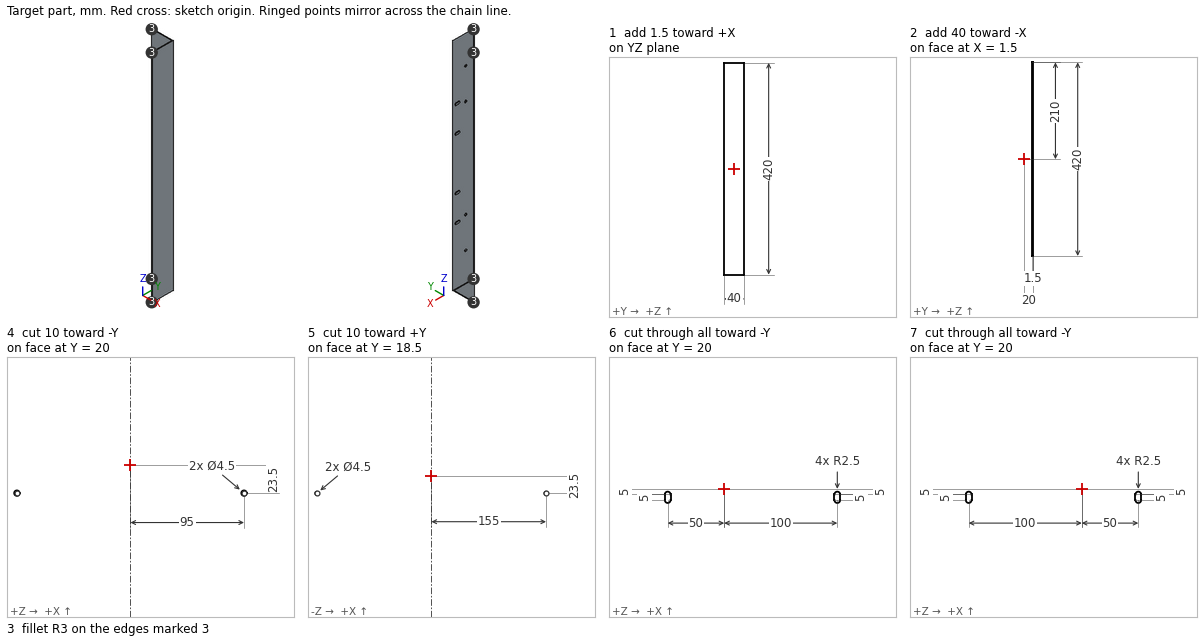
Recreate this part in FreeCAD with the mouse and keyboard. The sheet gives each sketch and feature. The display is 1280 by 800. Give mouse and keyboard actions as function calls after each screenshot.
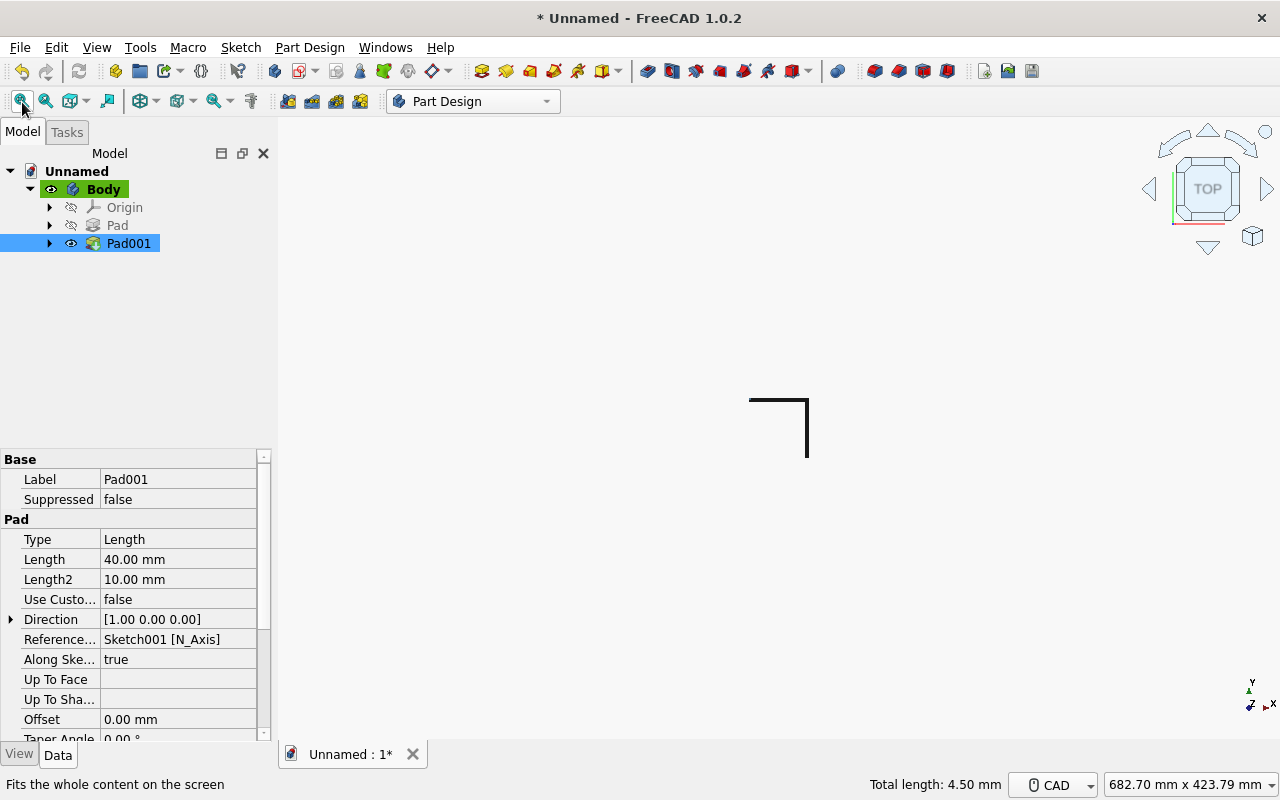
click(22, 102)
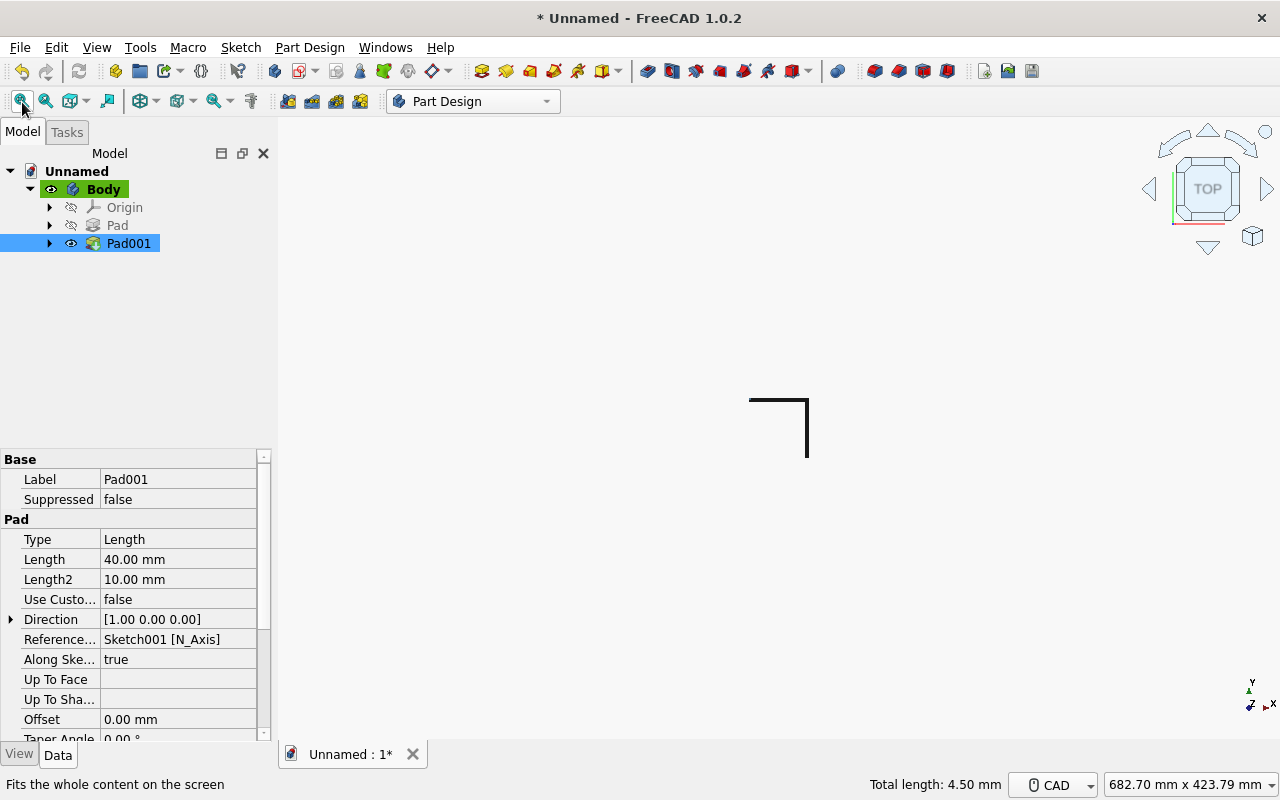
scroll(807, 456, up, 15)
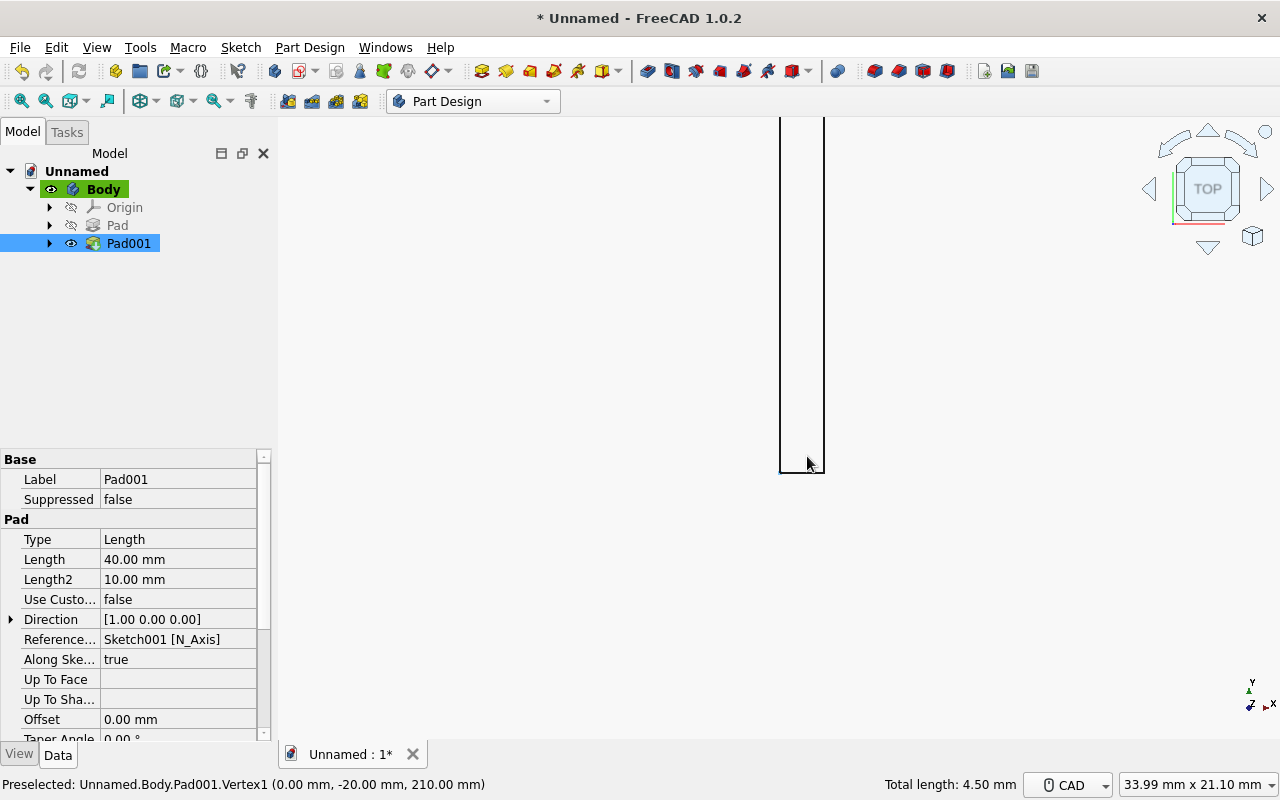
click(802, 472, ctrl)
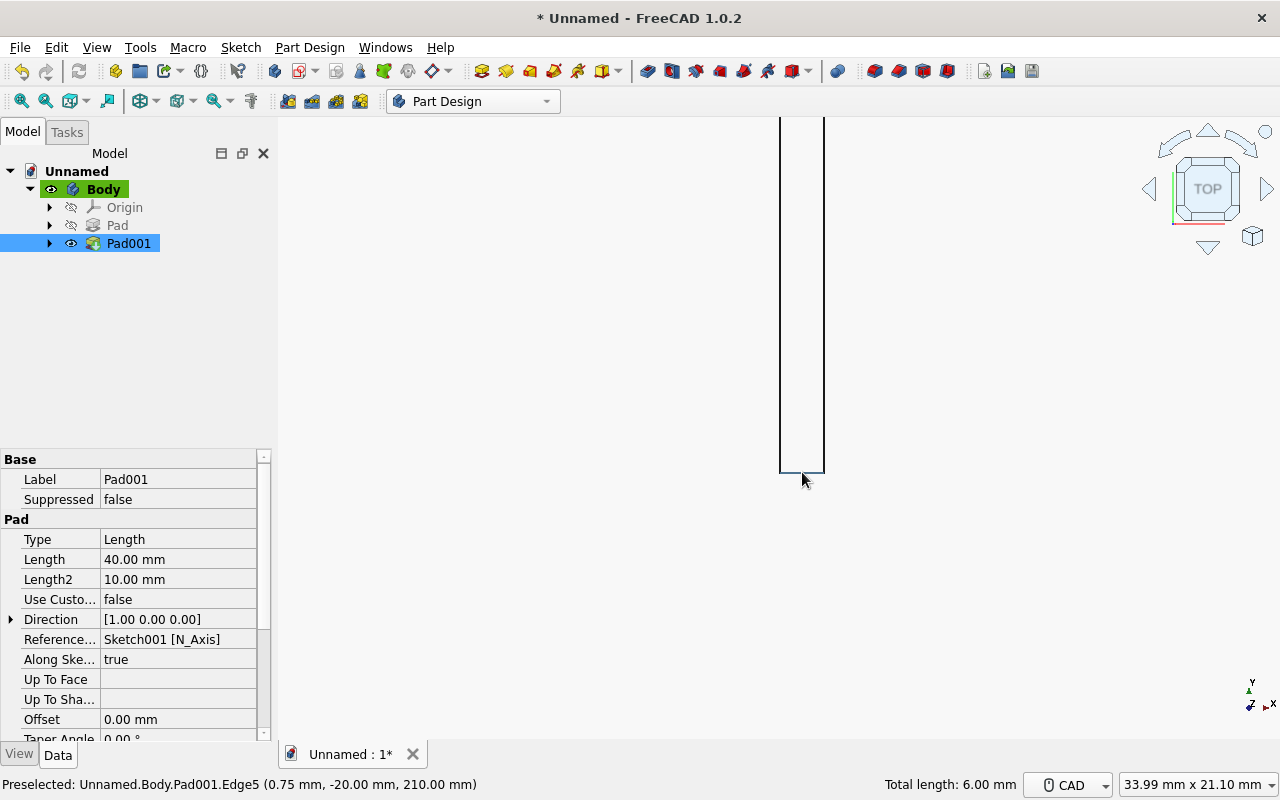
key(v)
key(1)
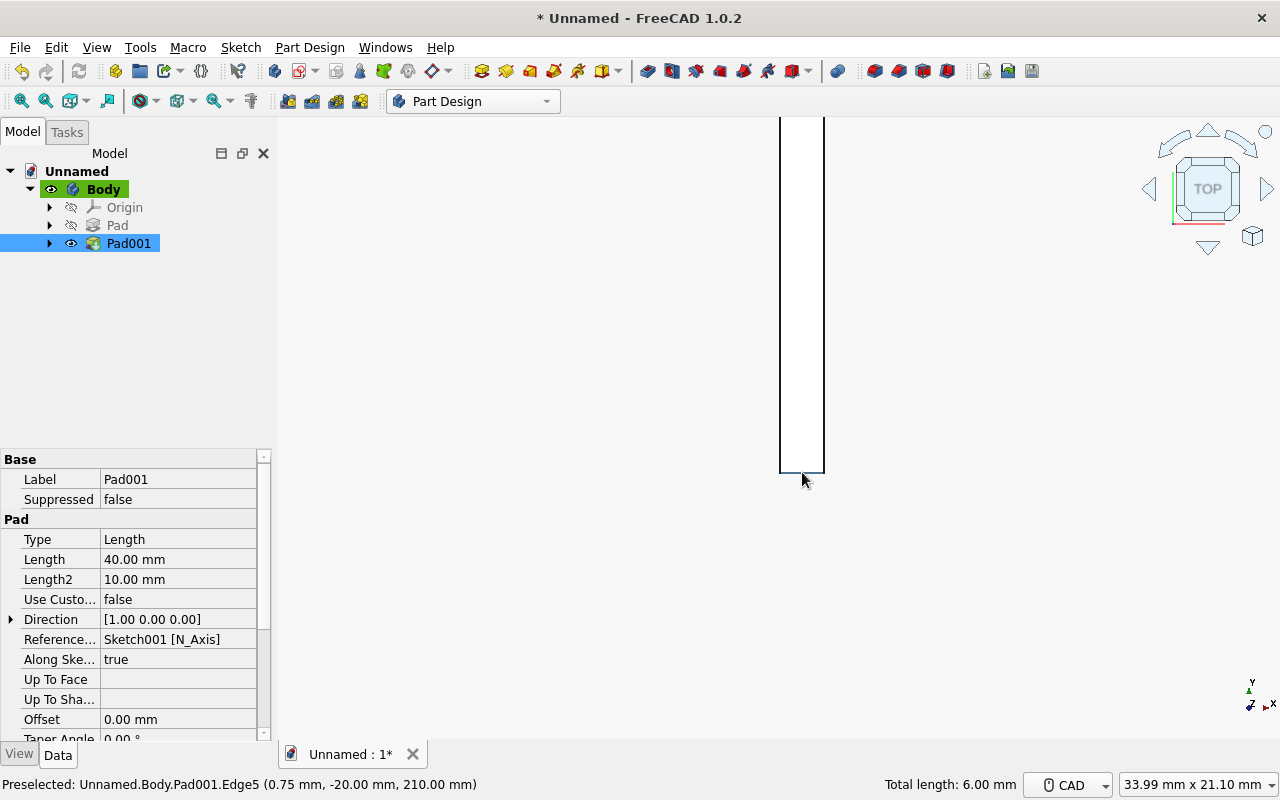
click(876, 72)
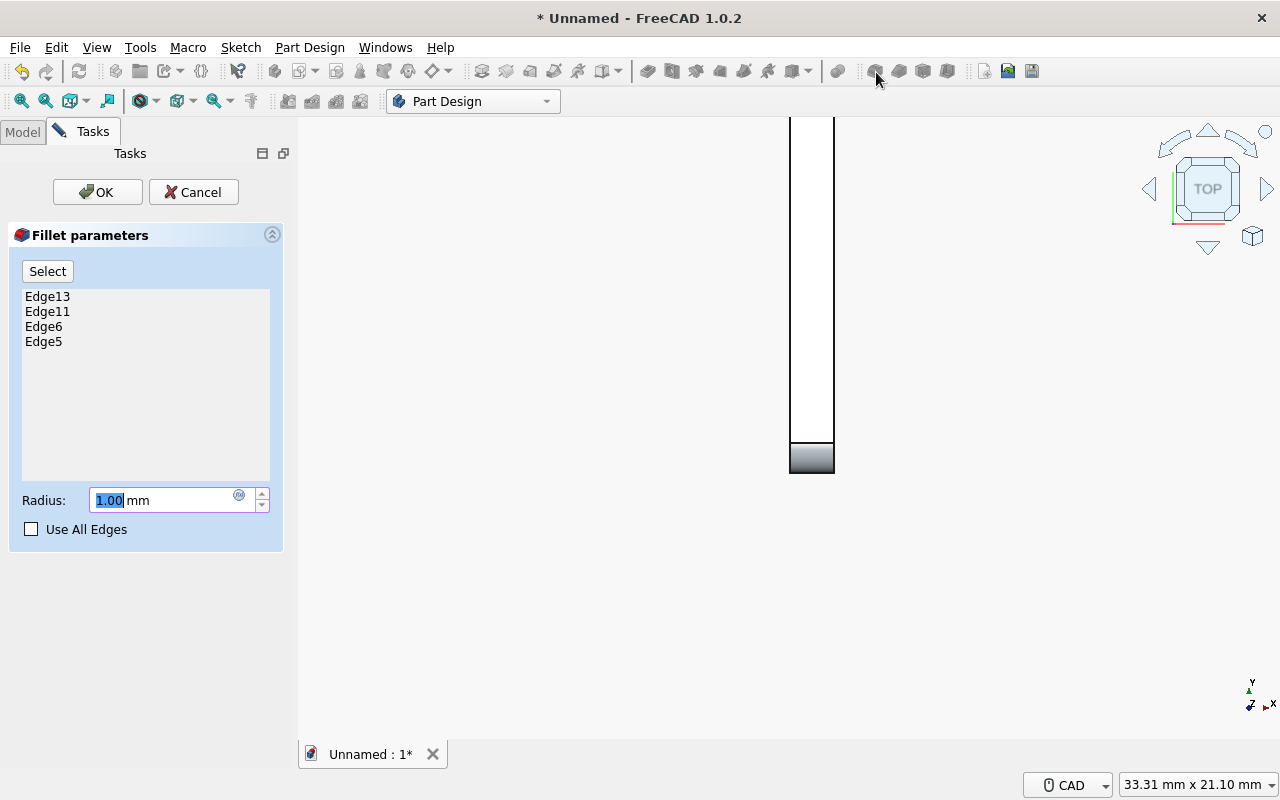
text(3)
key(Tab)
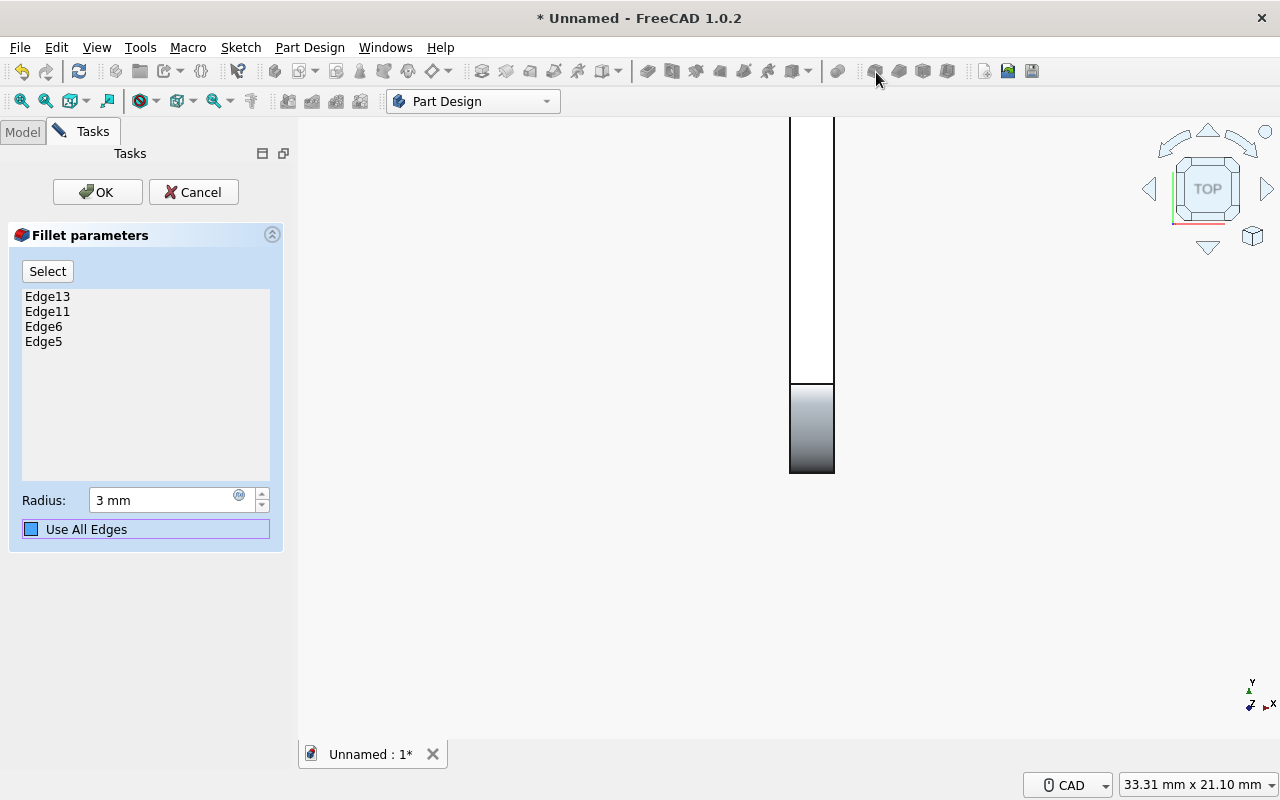
click(98, 192)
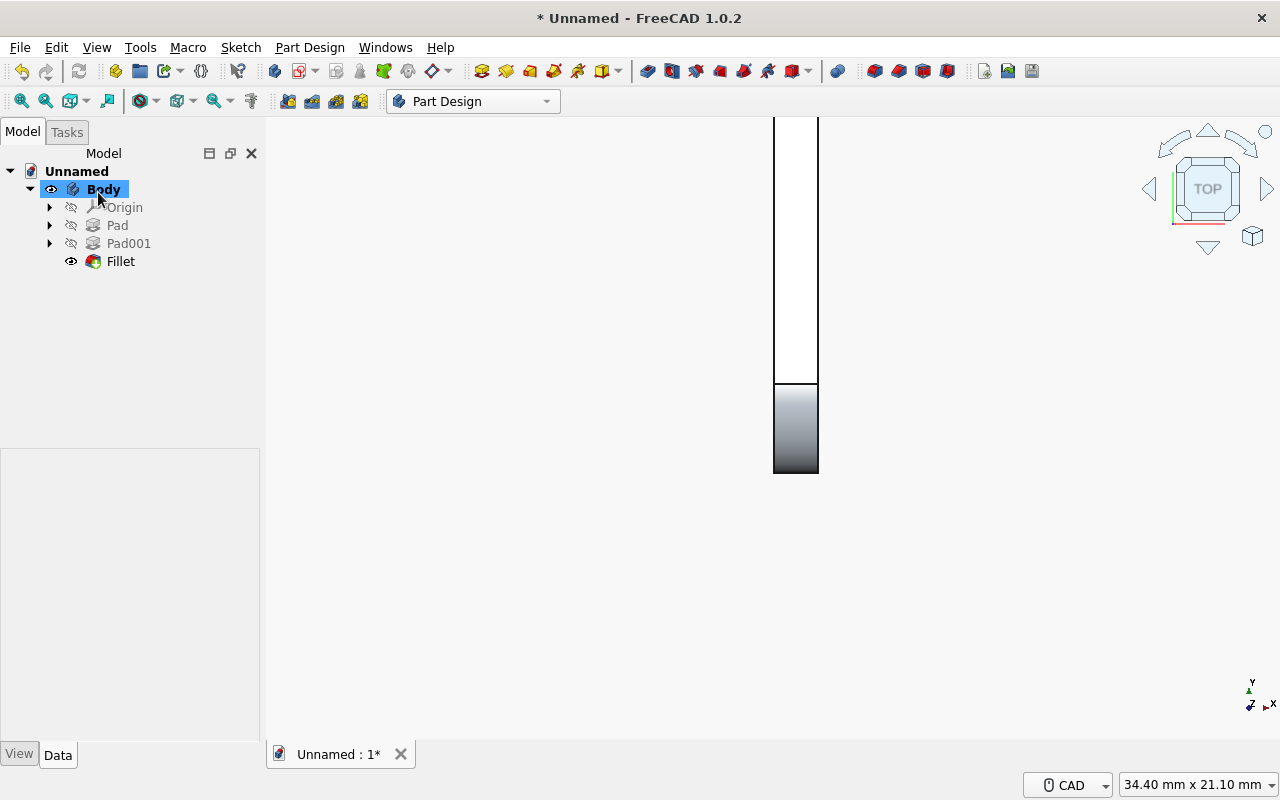
click(22, 102)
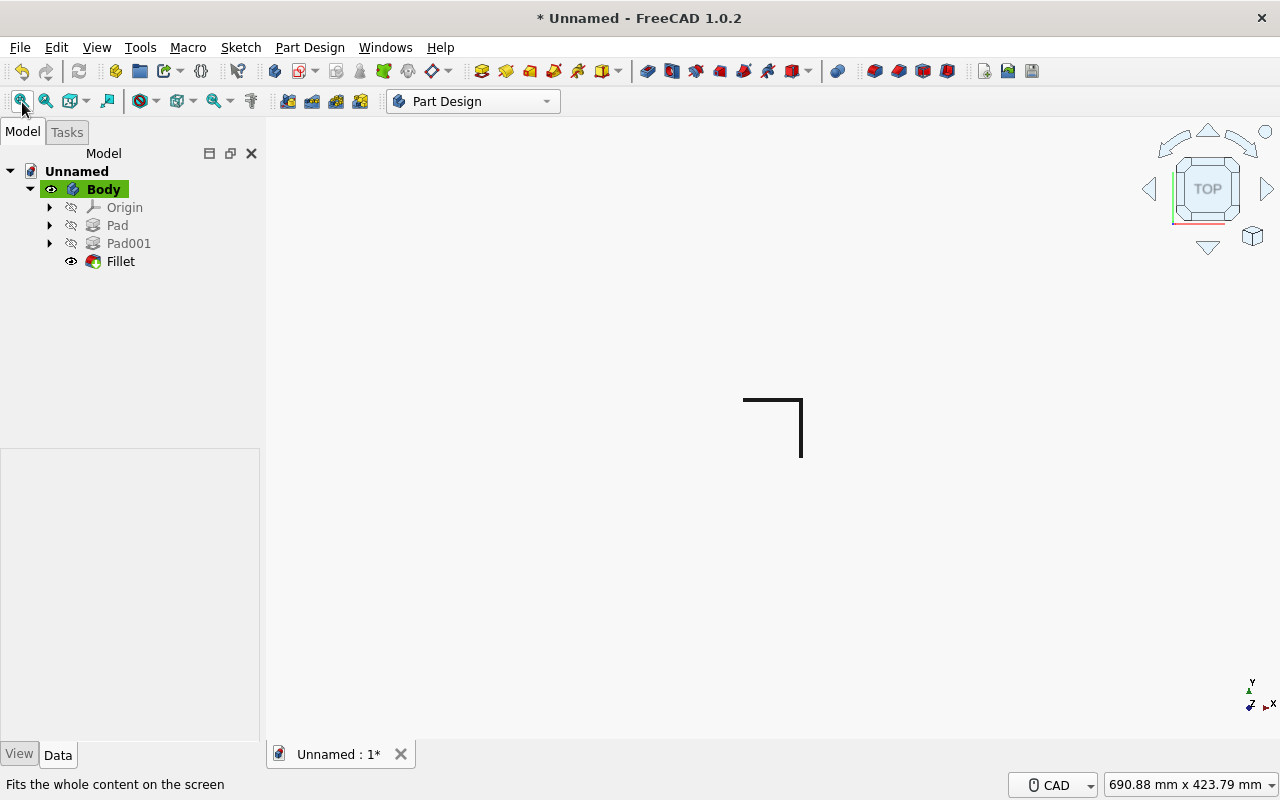
key(4)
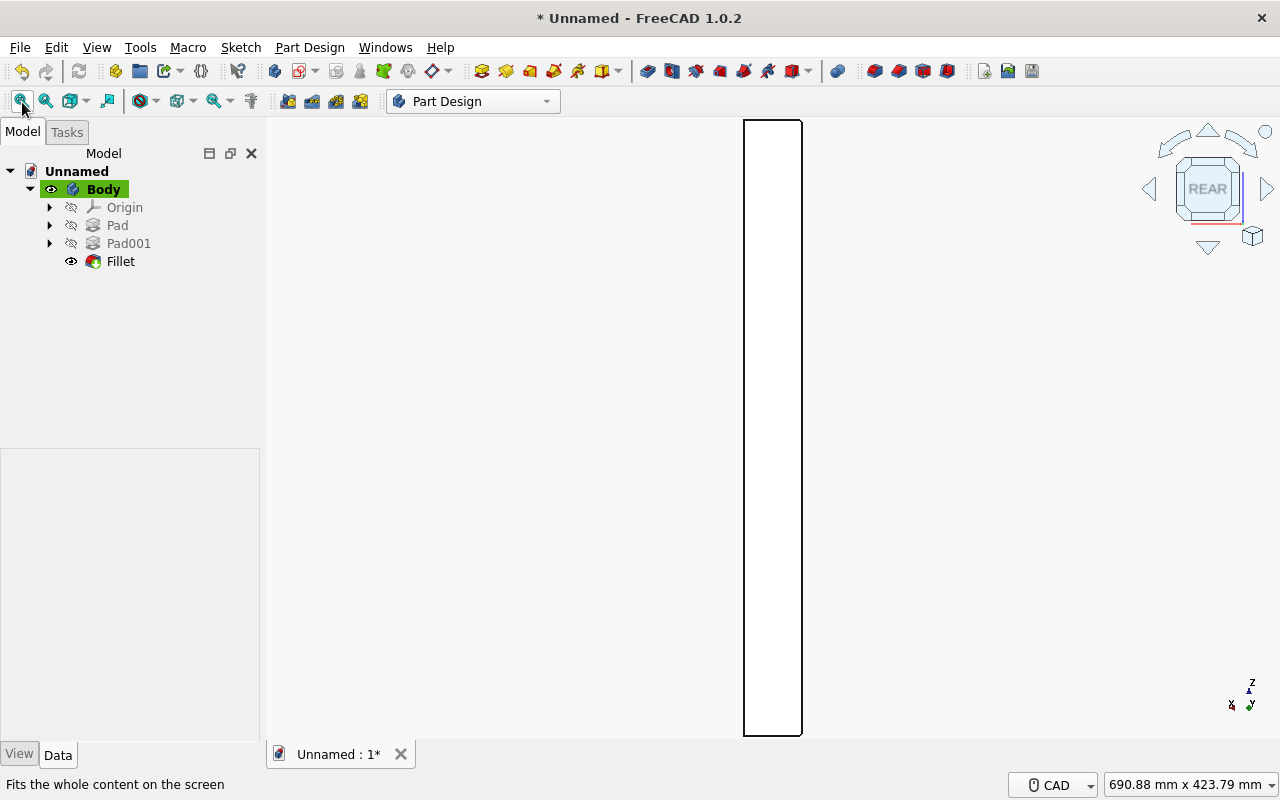
click(773, 603)